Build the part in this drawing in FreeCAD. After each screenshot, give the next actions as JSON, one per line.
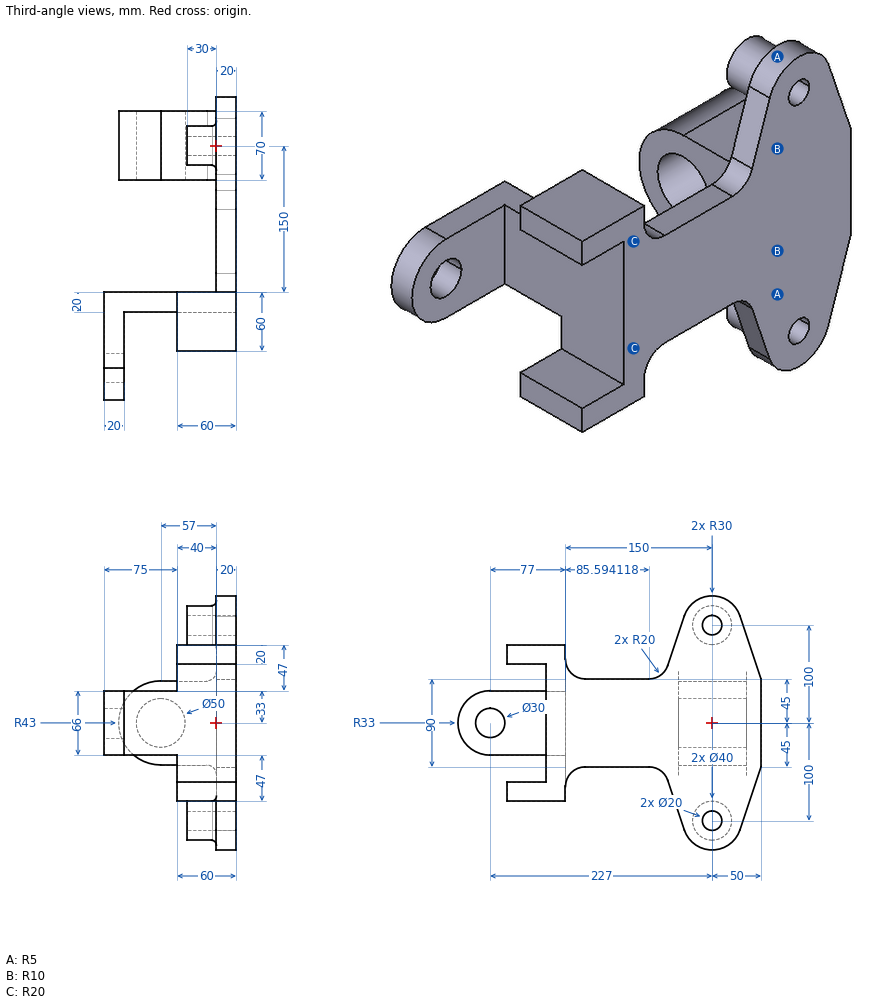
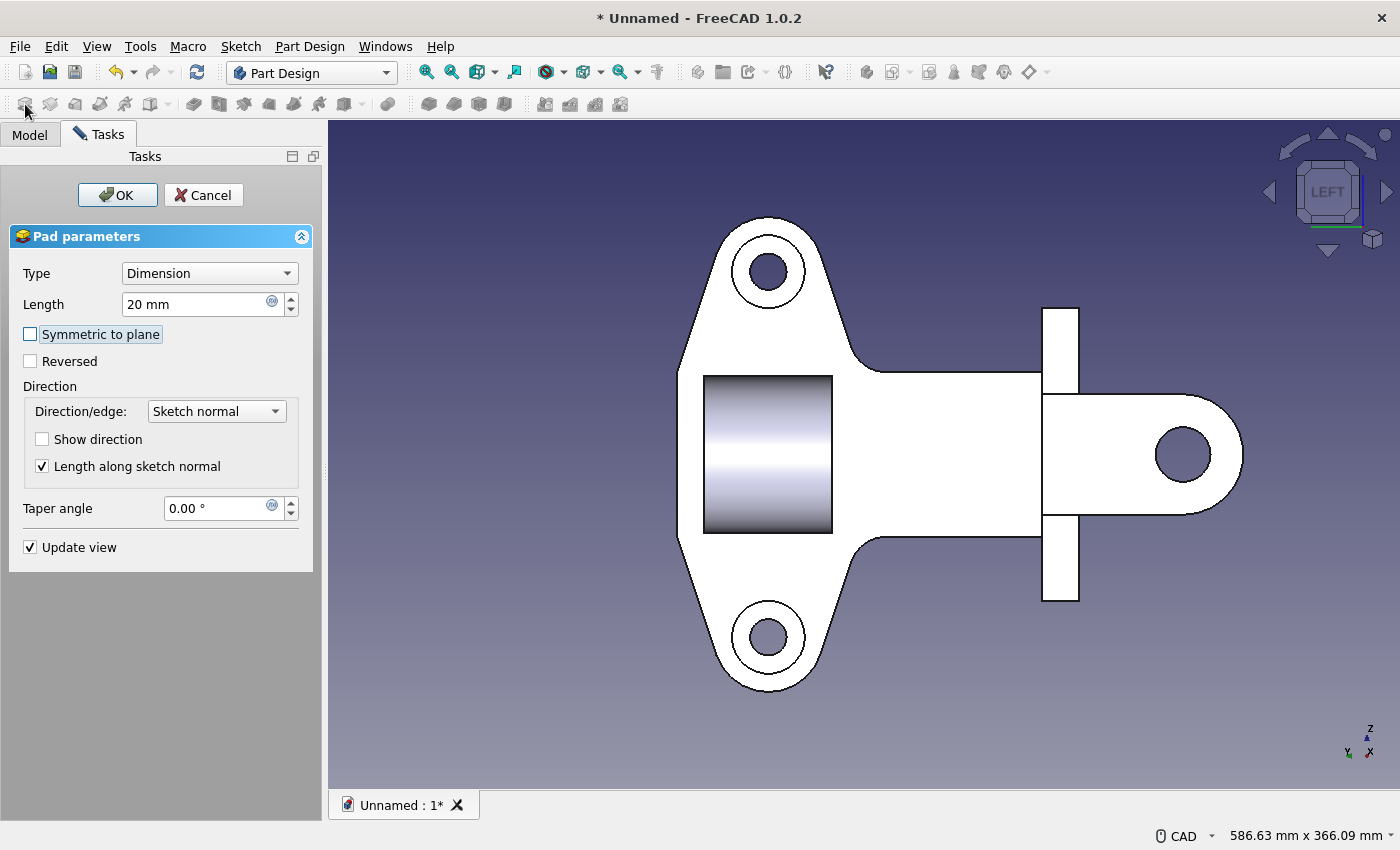
{"action": "left_click", "coordinate": [31, 361]}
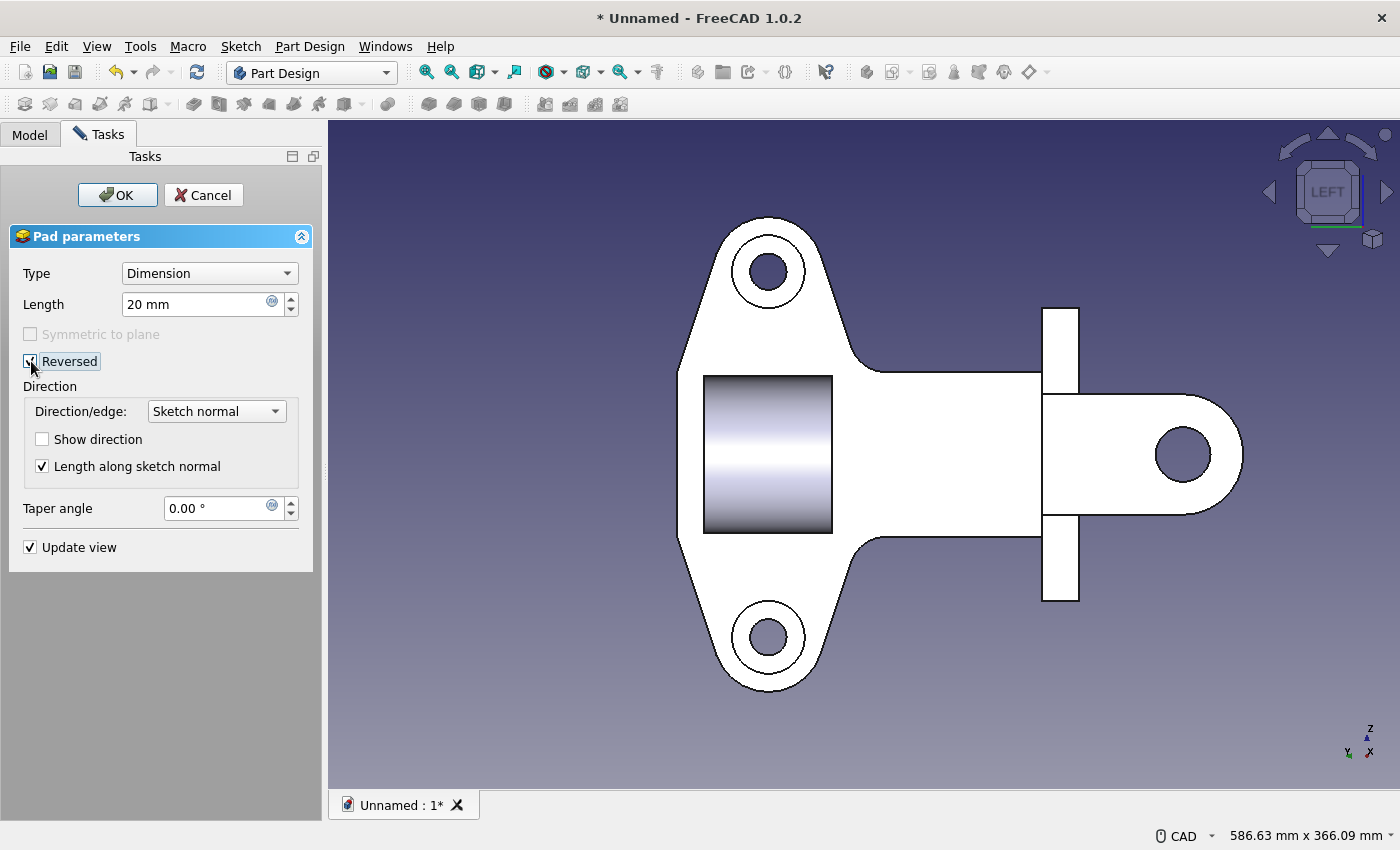
{"action": "left_click", "coordinate": [118, 195]}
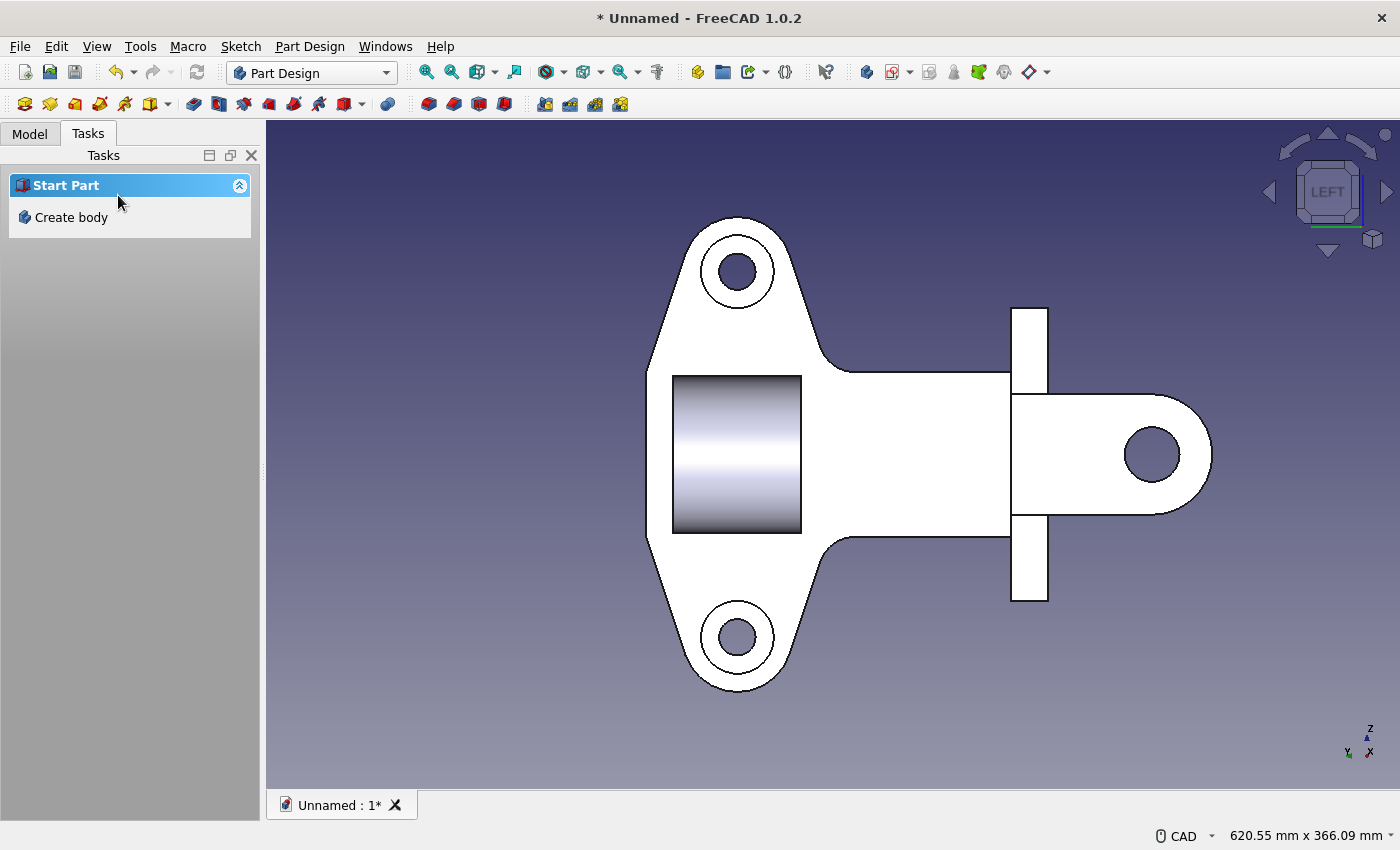
{"action": "key", "text": "0"}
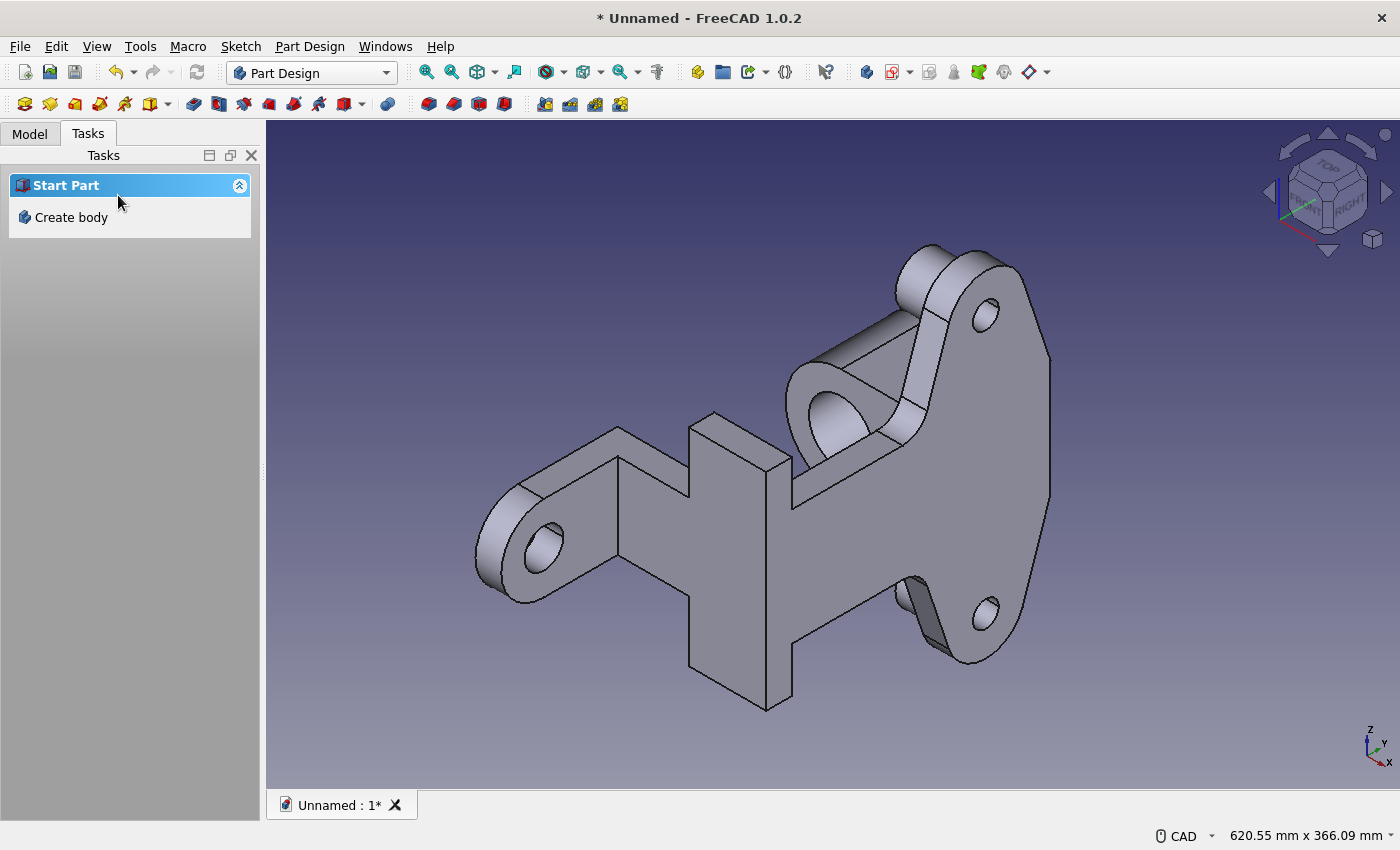
{"action": "key", "text": "v f"}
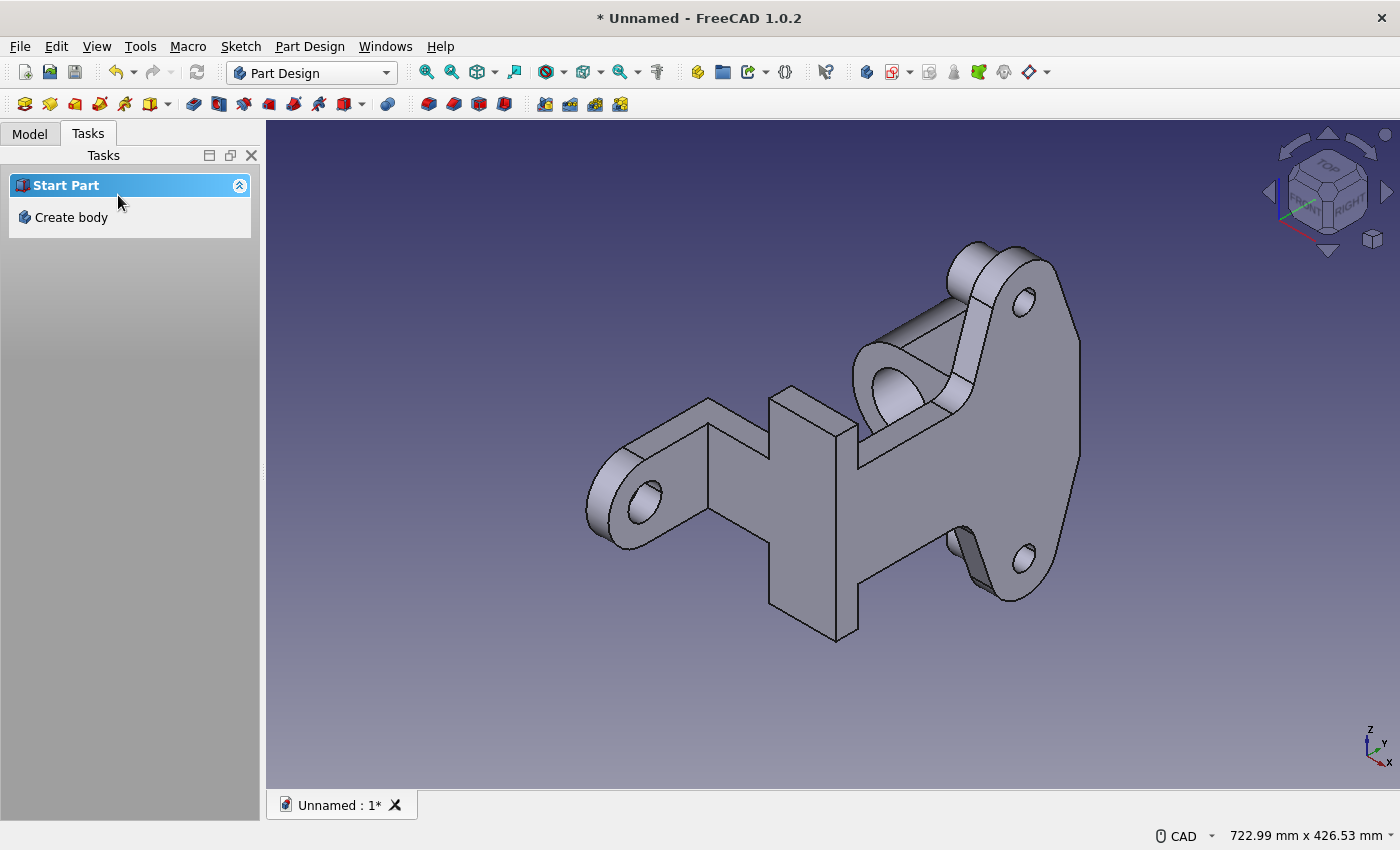
{"action": "left_click", "coordinate": [823, 416]}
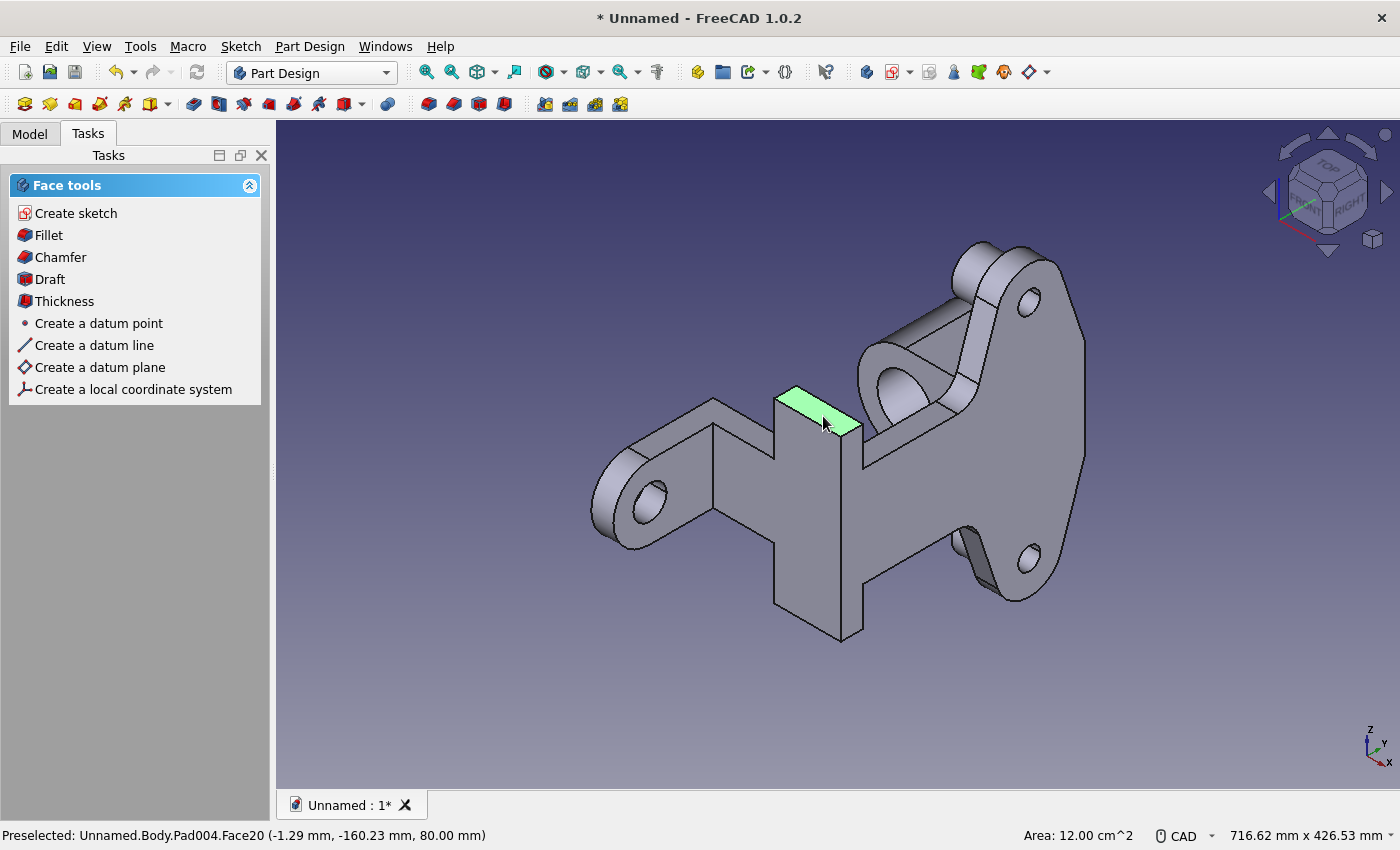
{"action": "left_click", "coordinate": [892, 72]}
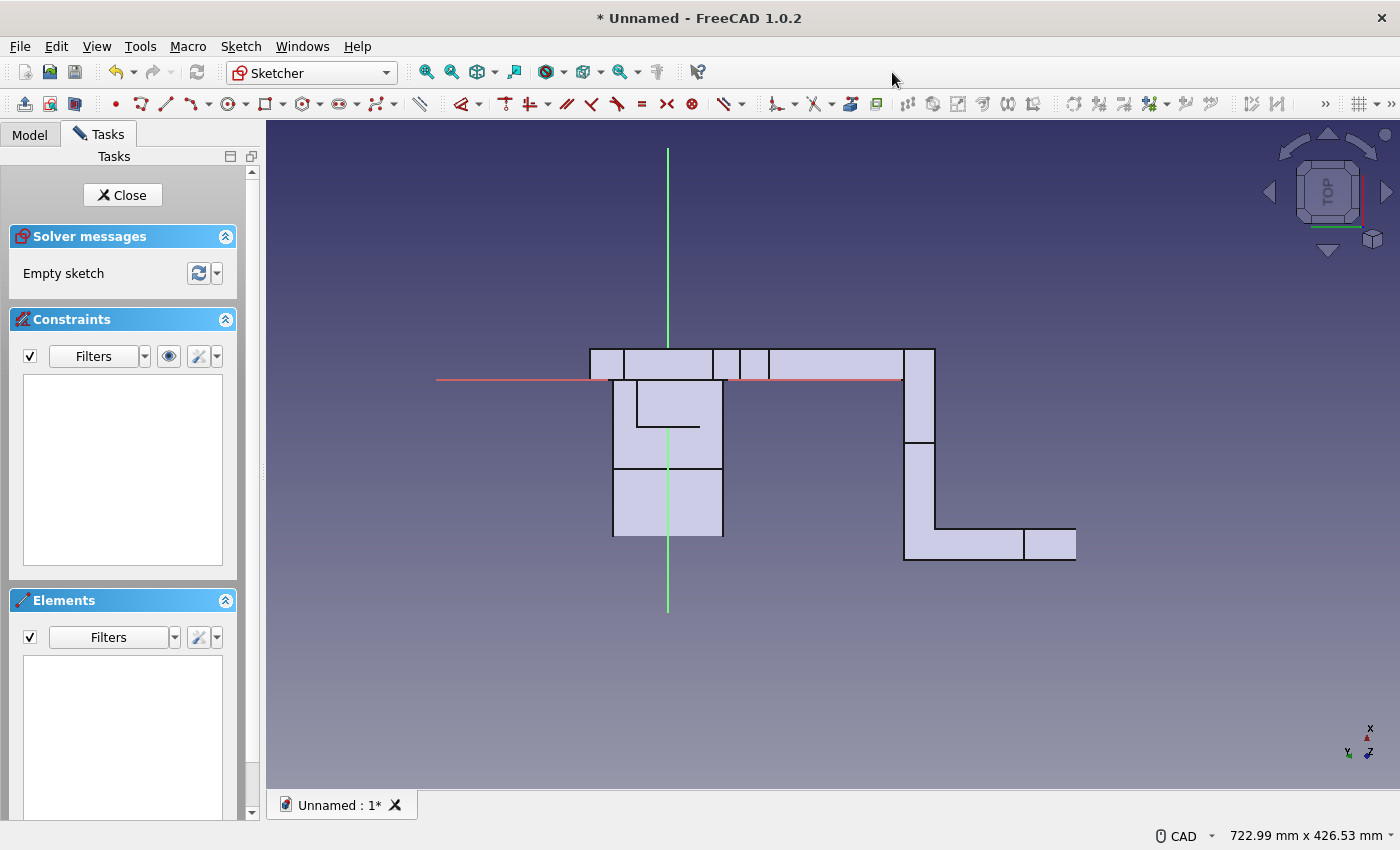
{"action": "scroll", "coordinate": [998, 381], "scroll_direction": "up", "scroll_amount": 8}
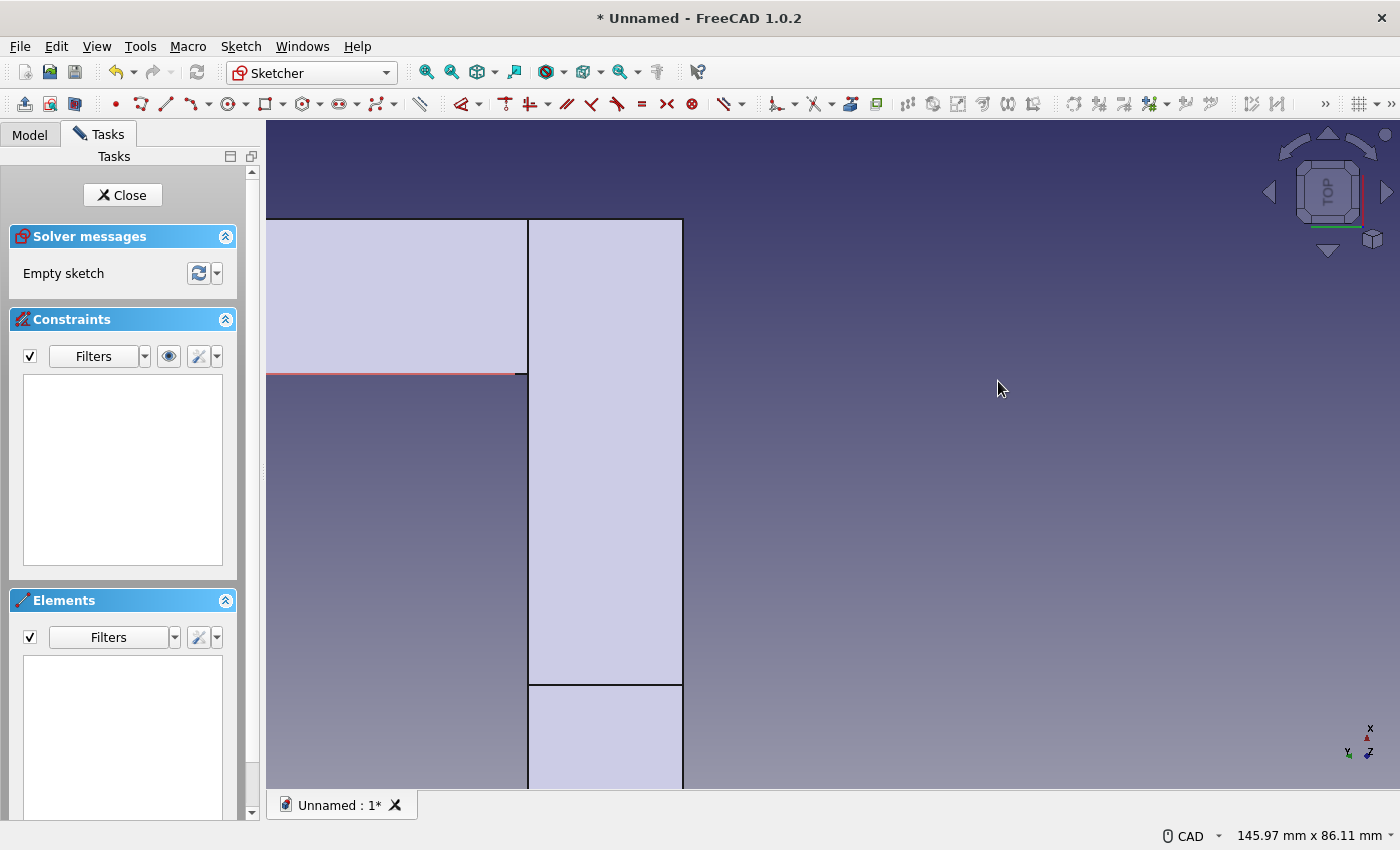
{"action": "left_click", "coordinate": [264, 104]}